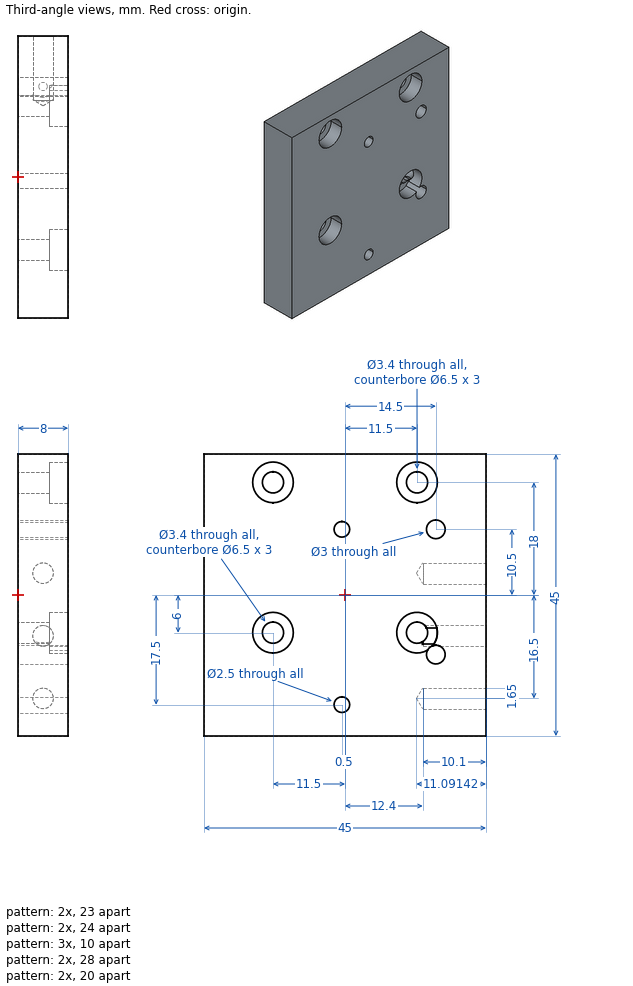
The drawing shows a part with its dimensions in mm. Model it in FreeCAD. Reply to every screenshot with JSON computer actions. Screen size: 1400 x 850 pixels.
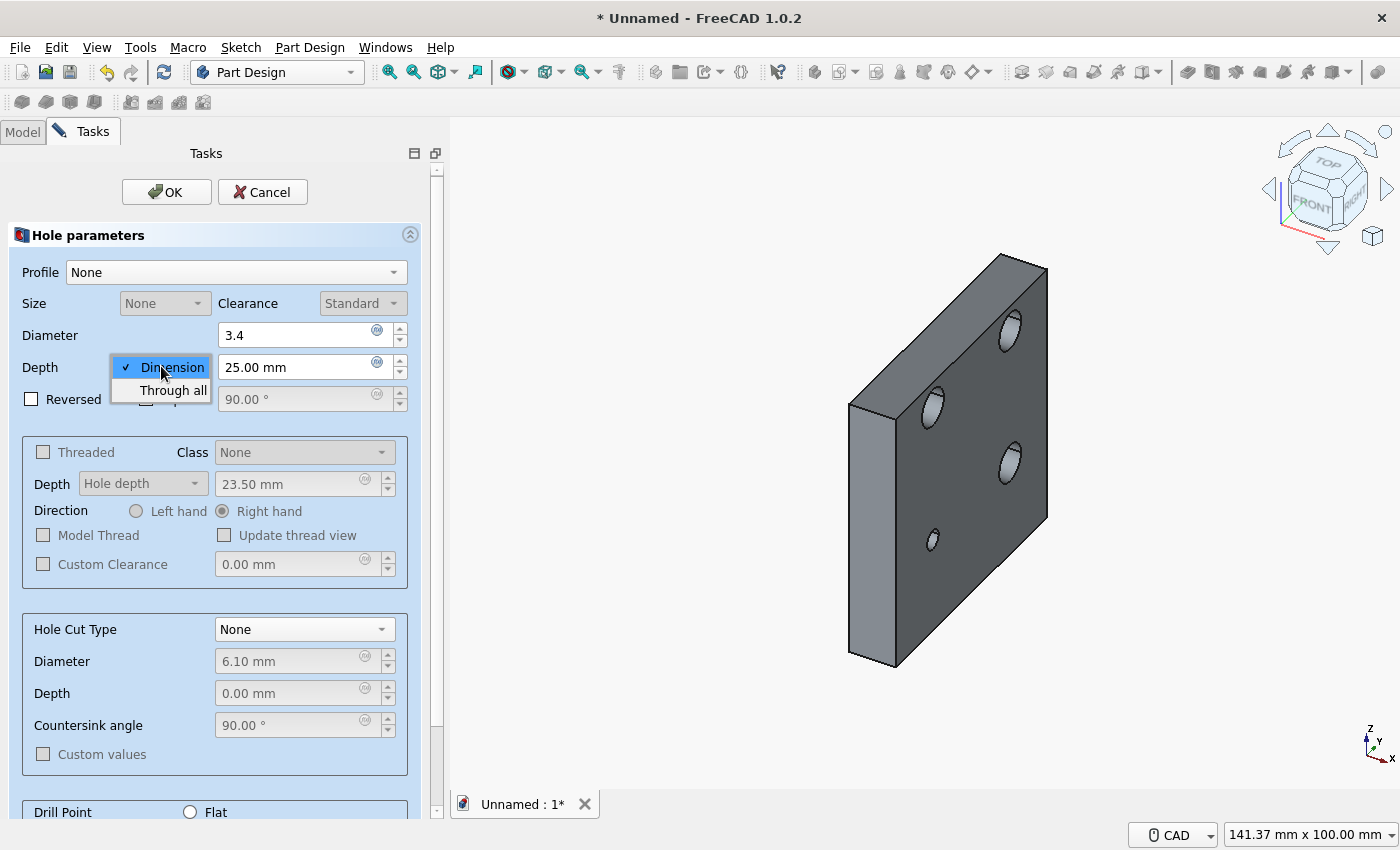
{"action": "left_click", "coordinate": [160, 390]}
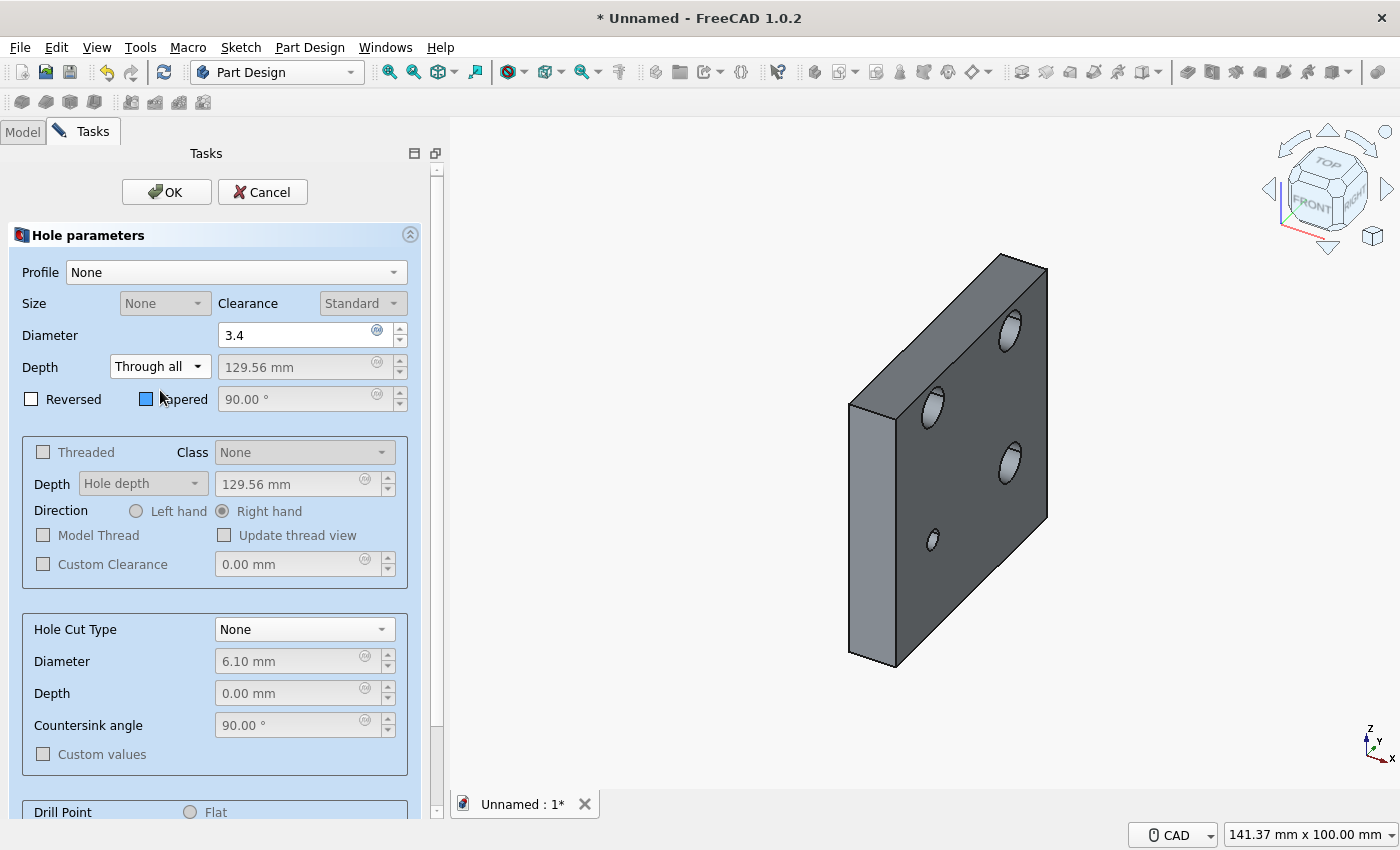
{"action": "left_click", "coordinate": [306, 630]}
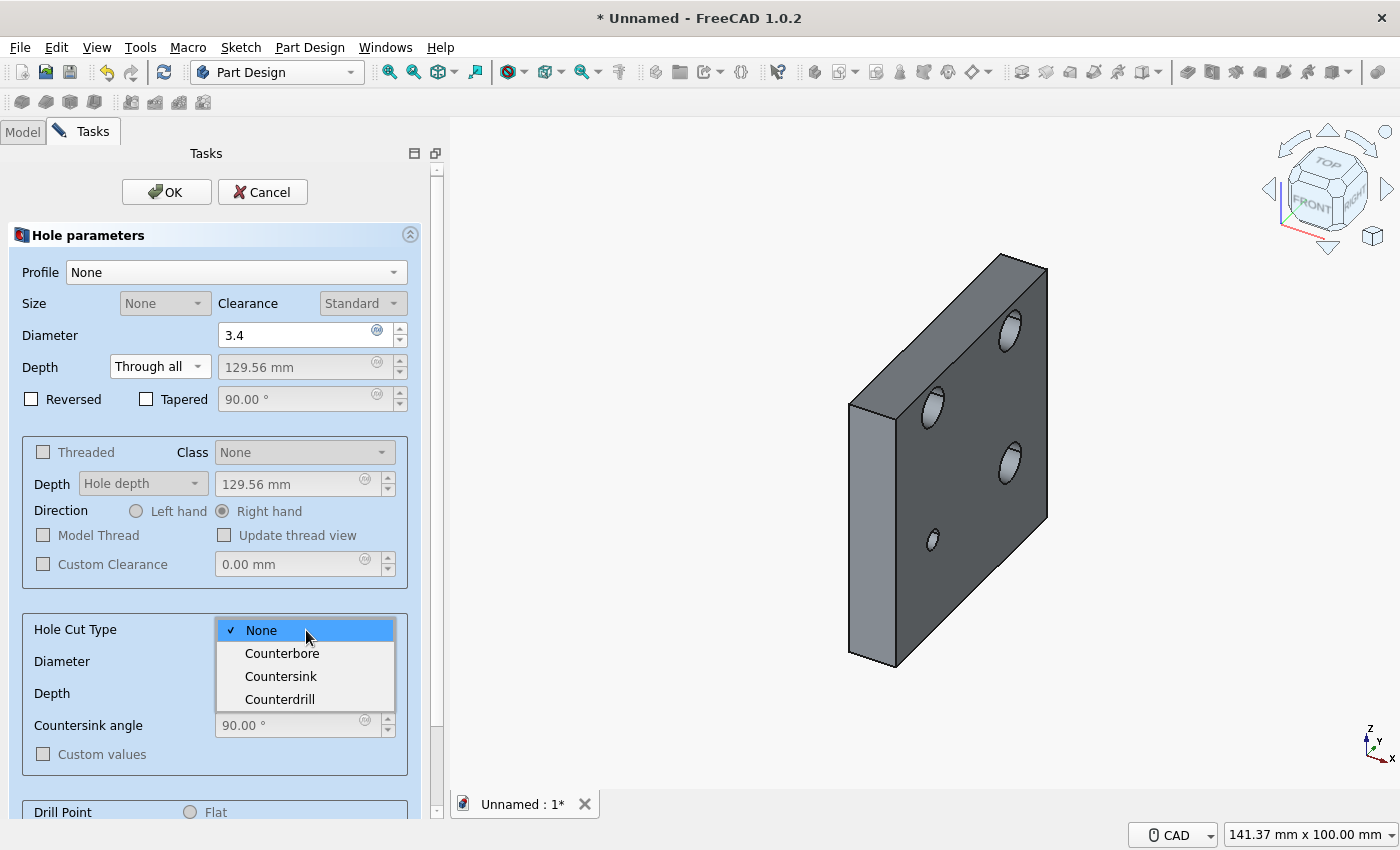
{"action": "left_click", "coordinate": [304, 654]}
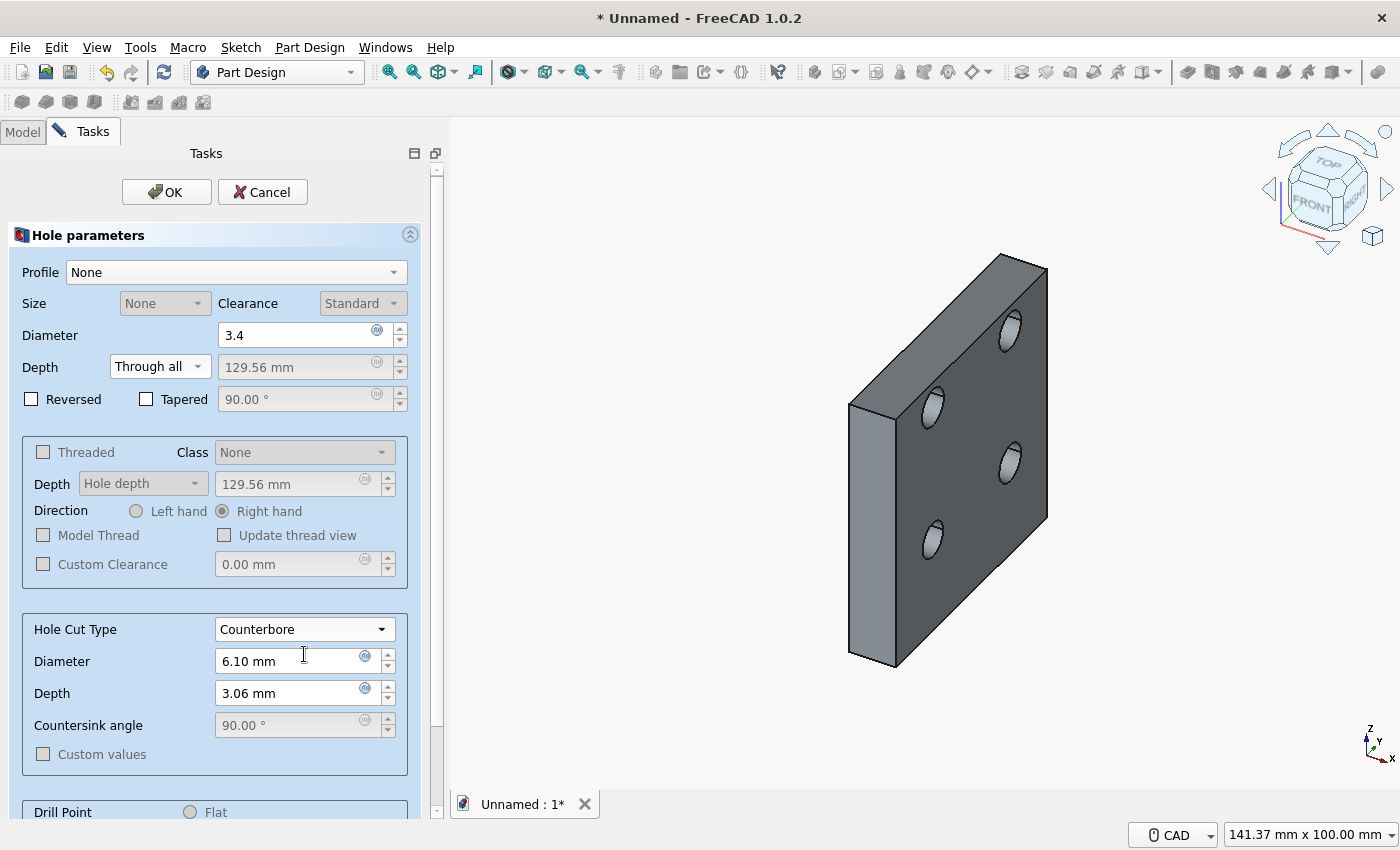
{"action": "triple_click", "coordinate": [298, 661]}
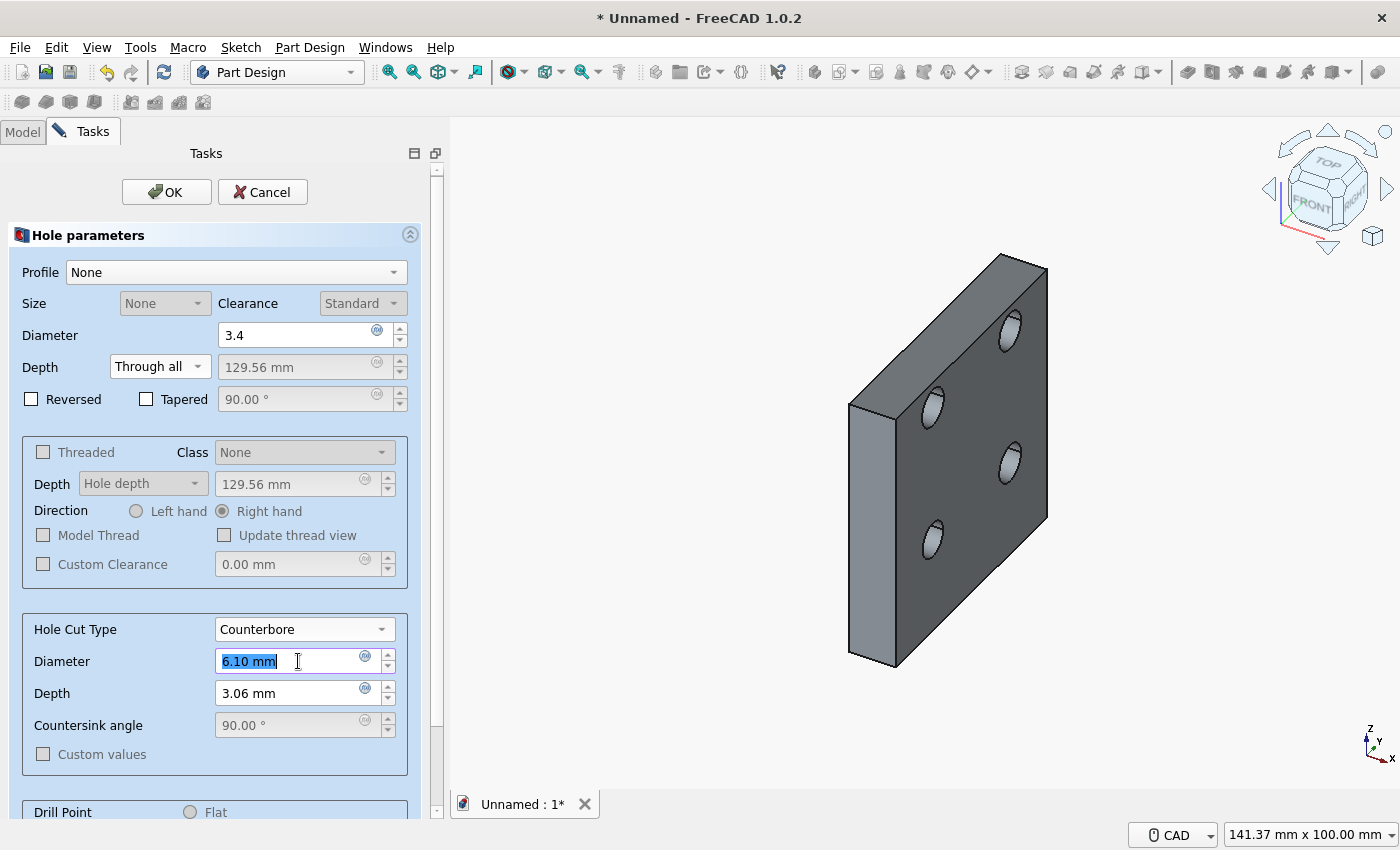
{"action": "type", "text": "6.5"}
{"action": "key", "text": "Tab"}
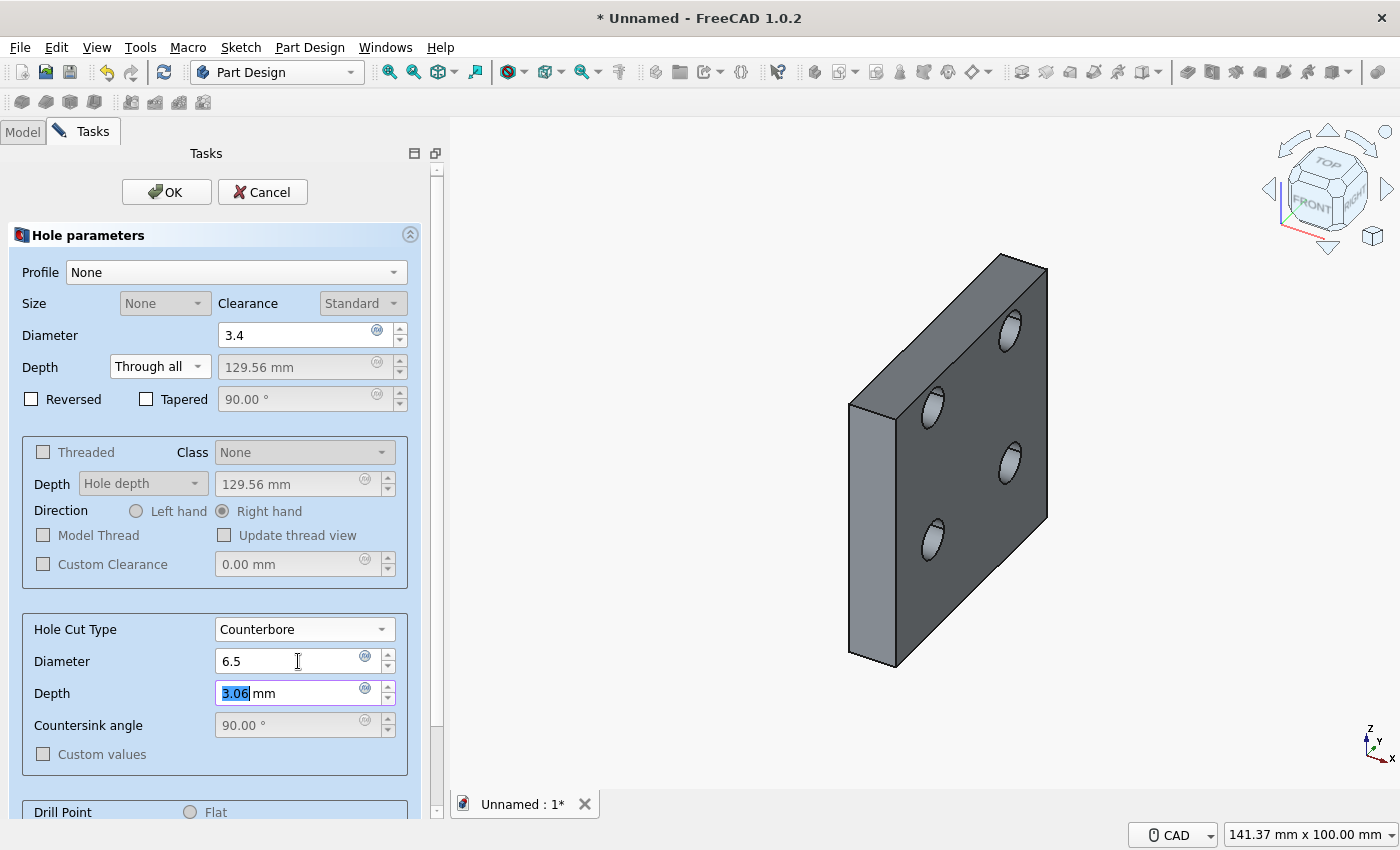
{"action": "type", "text": "3"}
{"action": "key", "text": "Tab"}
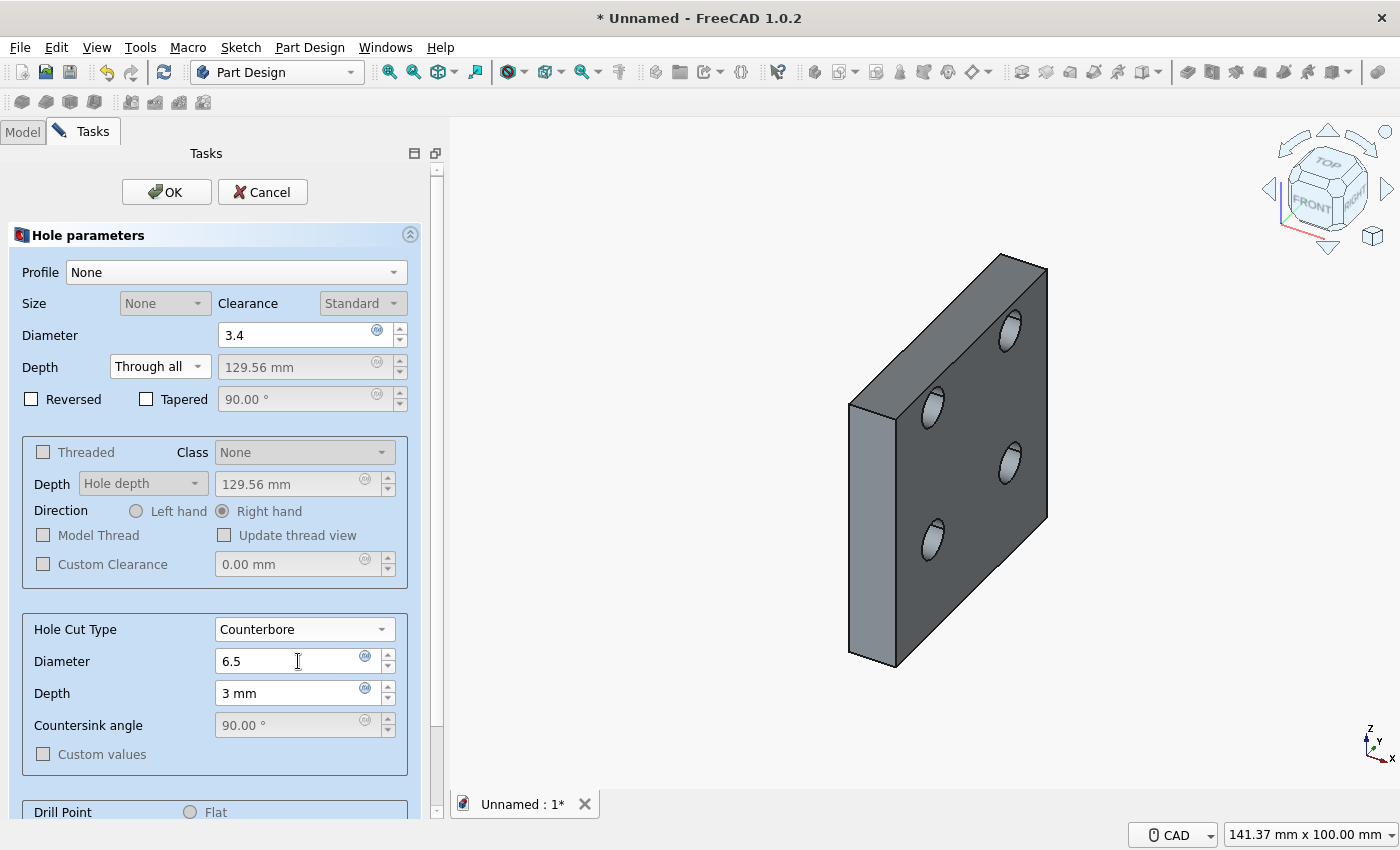
{"action": "left_click", "coordinate": [167, 192]}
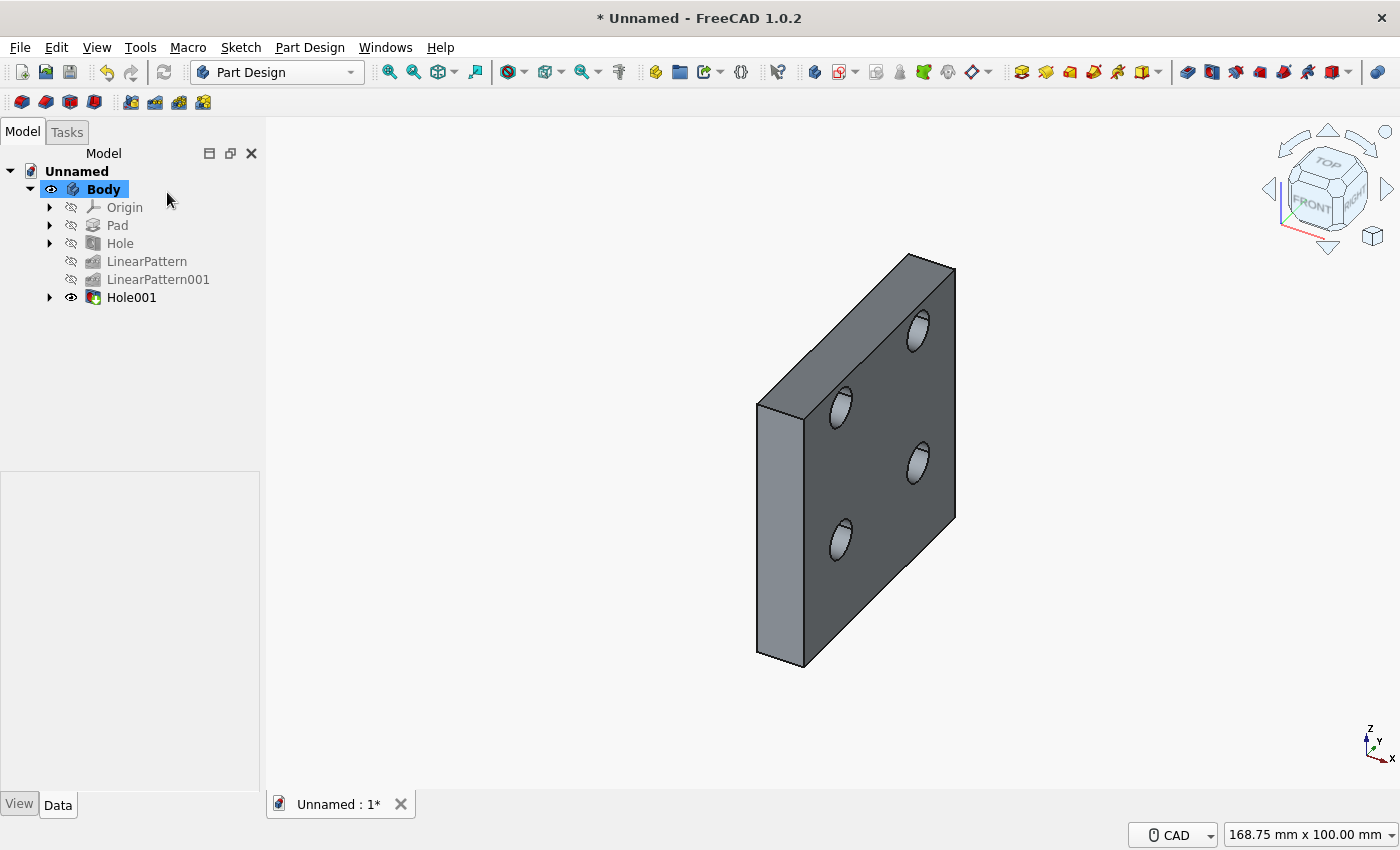
{"action": "left_click", "coordinate": [50, 207]}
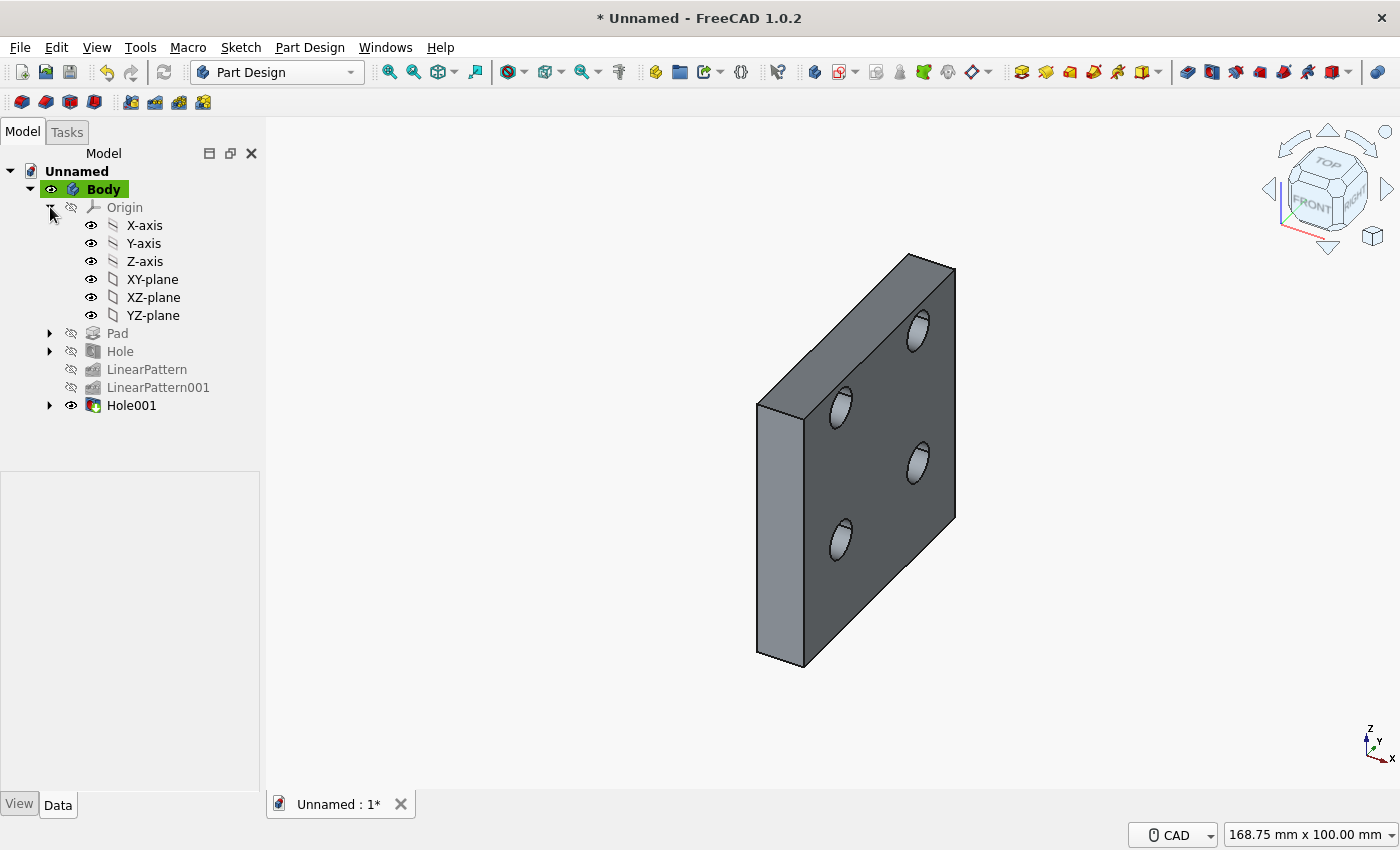
{"action": "left_click", "coordinate": [136, 315]}